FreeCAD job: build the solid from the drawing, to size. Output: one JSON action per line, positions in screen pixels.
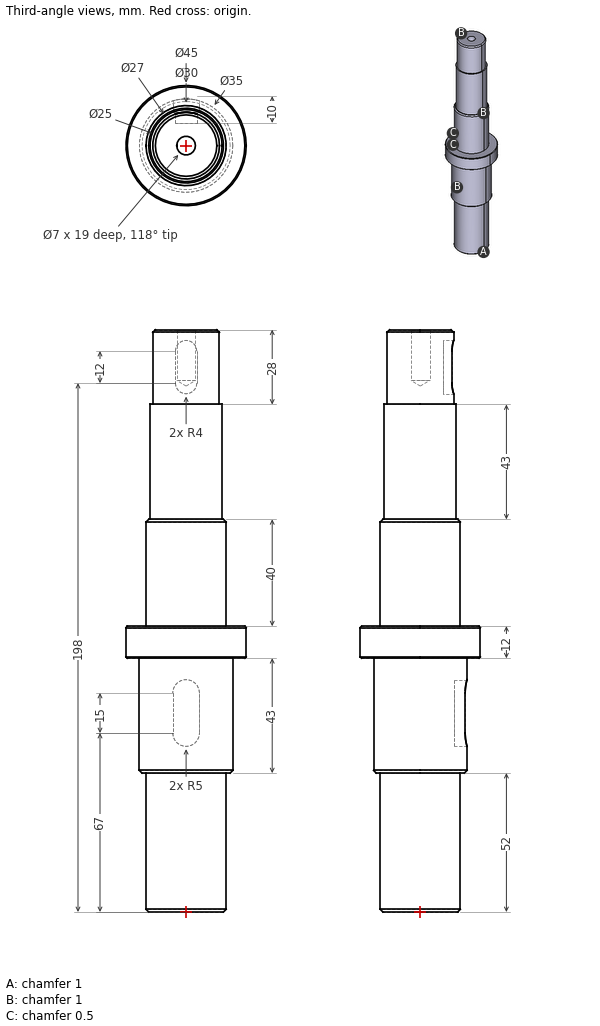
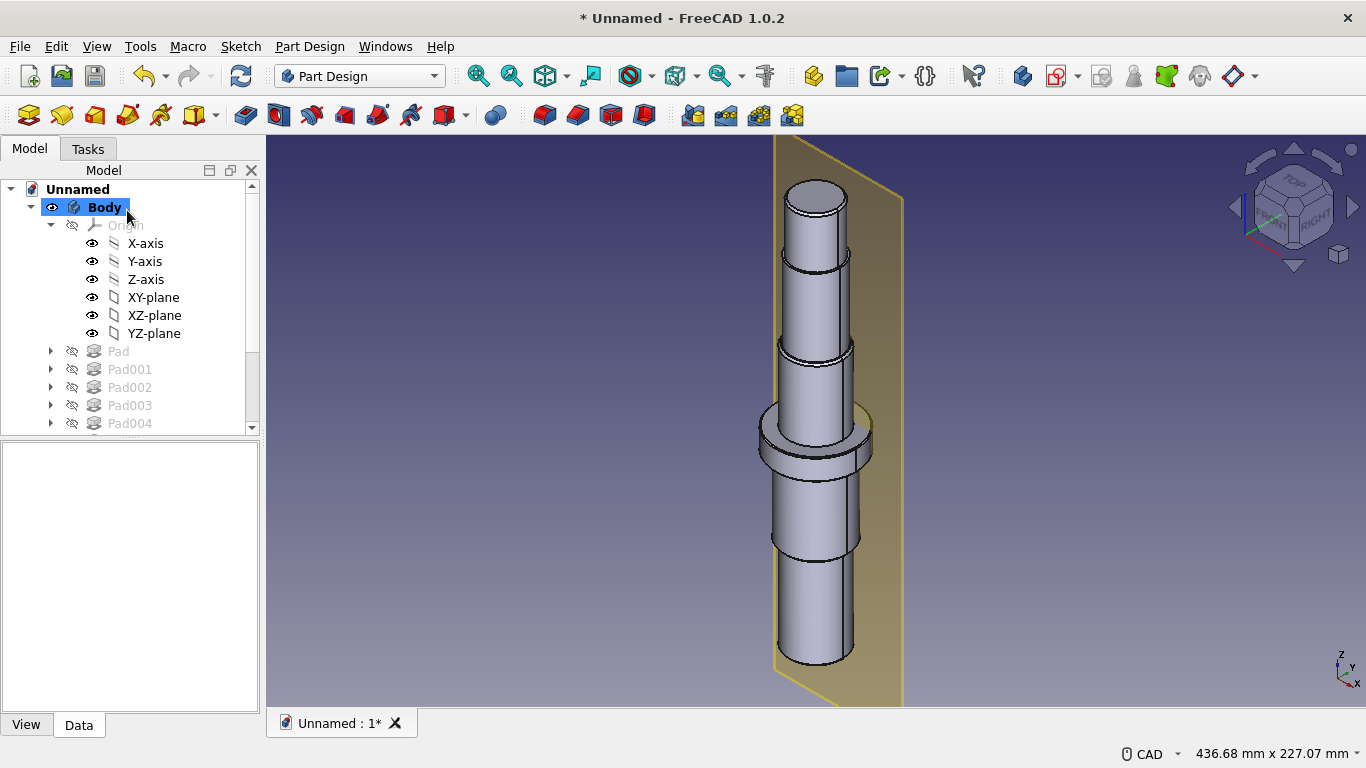
{"action": "scroll", "coordinate": [101, 311], "scroll_direction": "down", "scroll_amount": 3}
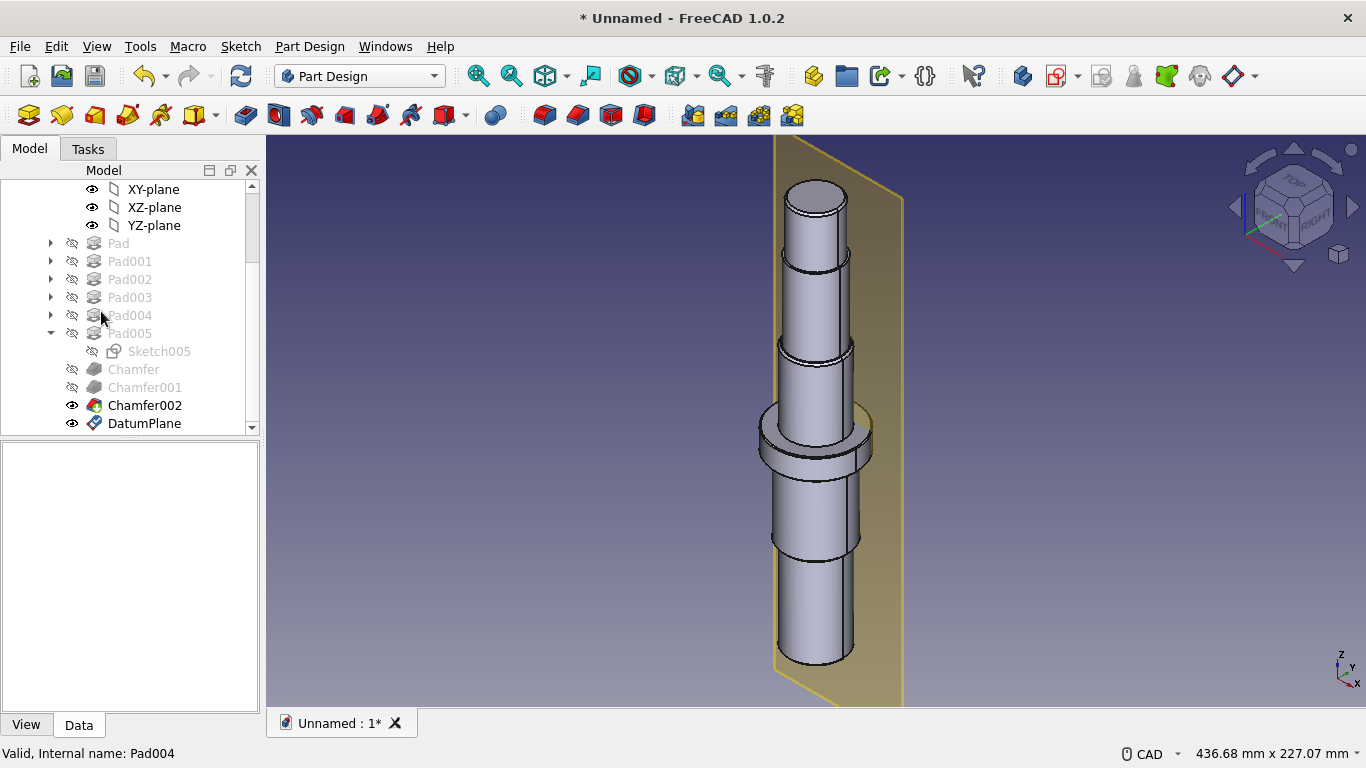
{"action": "left_click", "coordinate": [117, 423]}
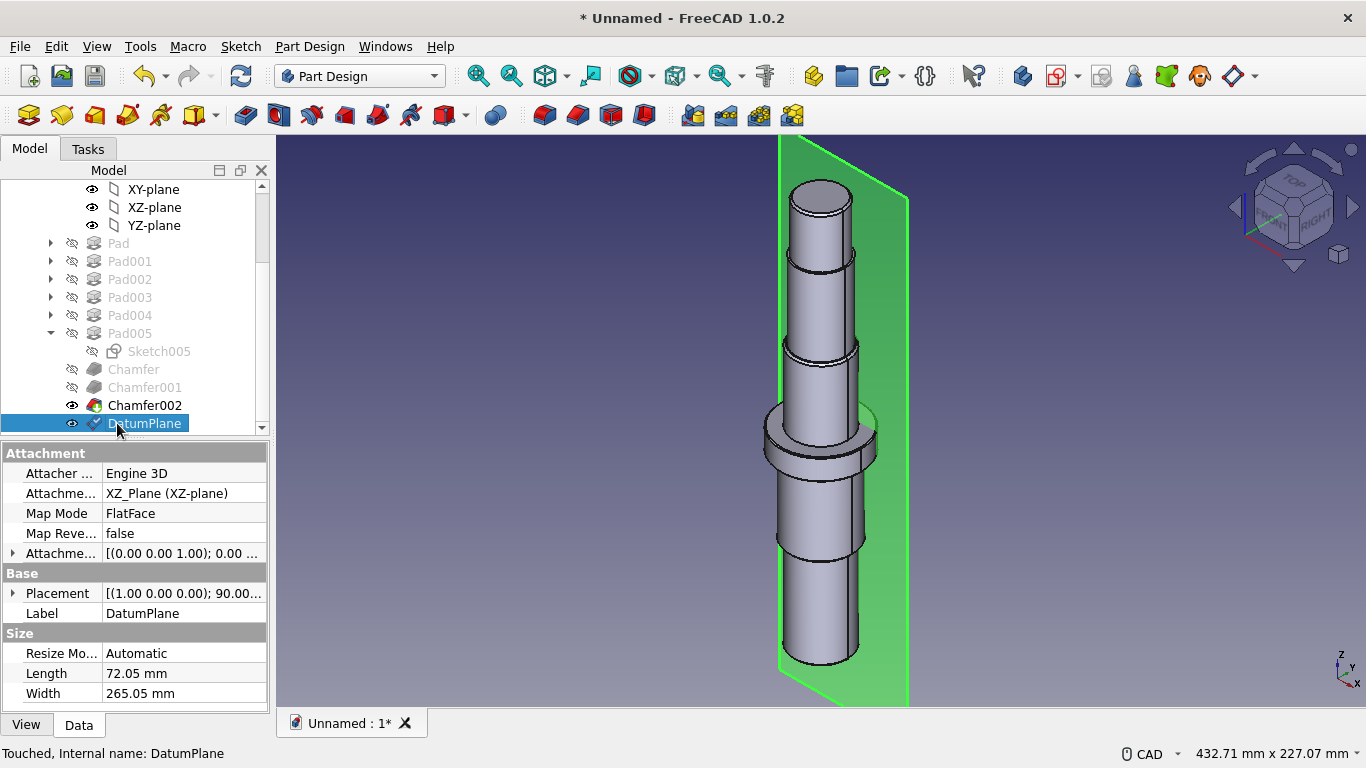
{"action": "left_click", "coordinate": [1056, 76]}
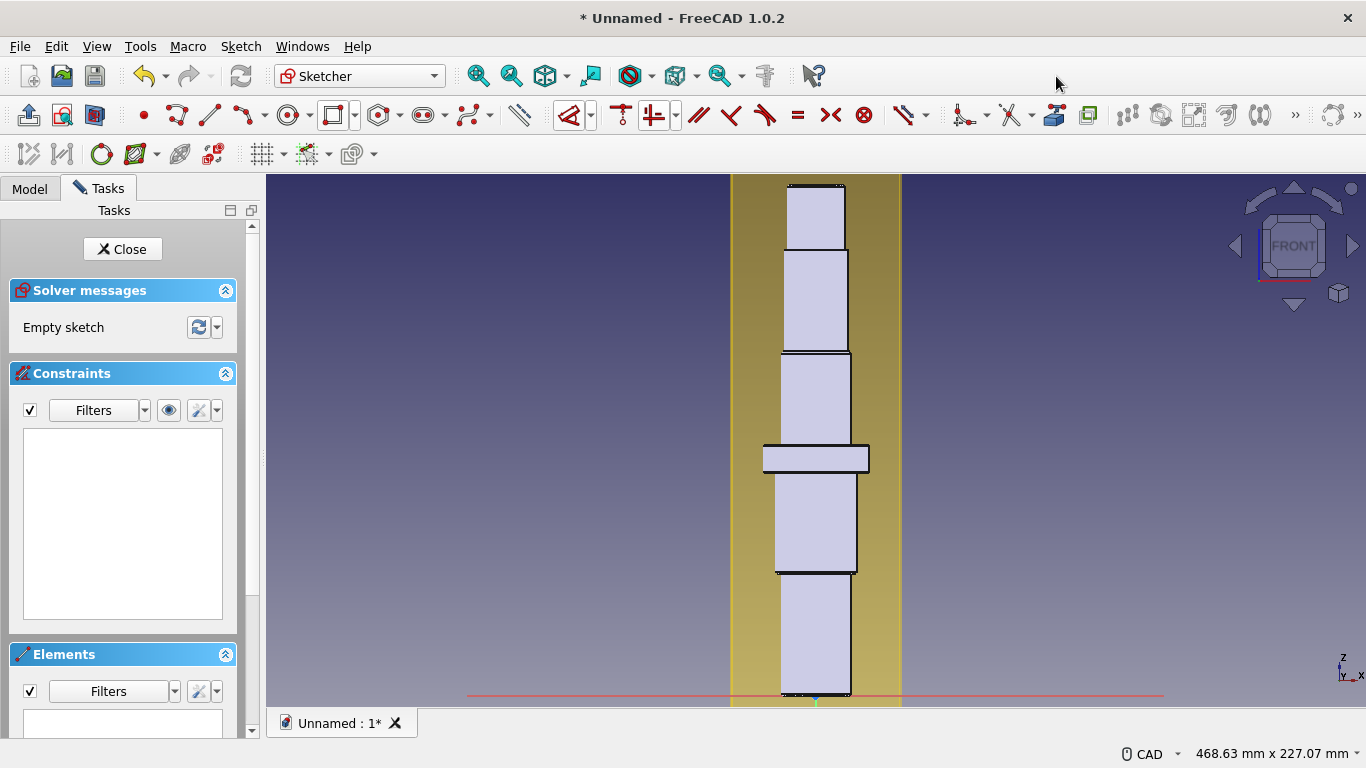
{"action": "left_click", "coordinate": [95, 116]}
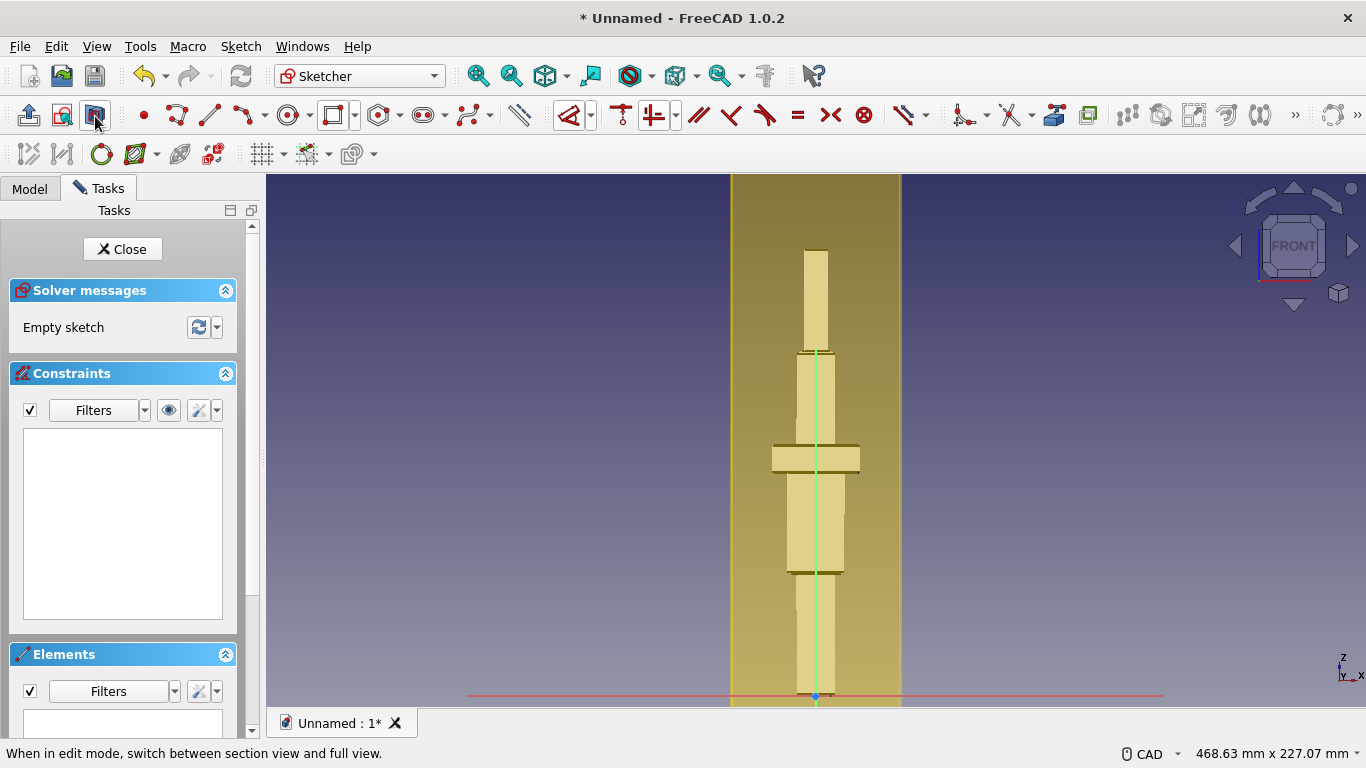
{"action": "scroll", "coordinate": [829, 538], "scroll_direction": "up", "scroll_amount": 9}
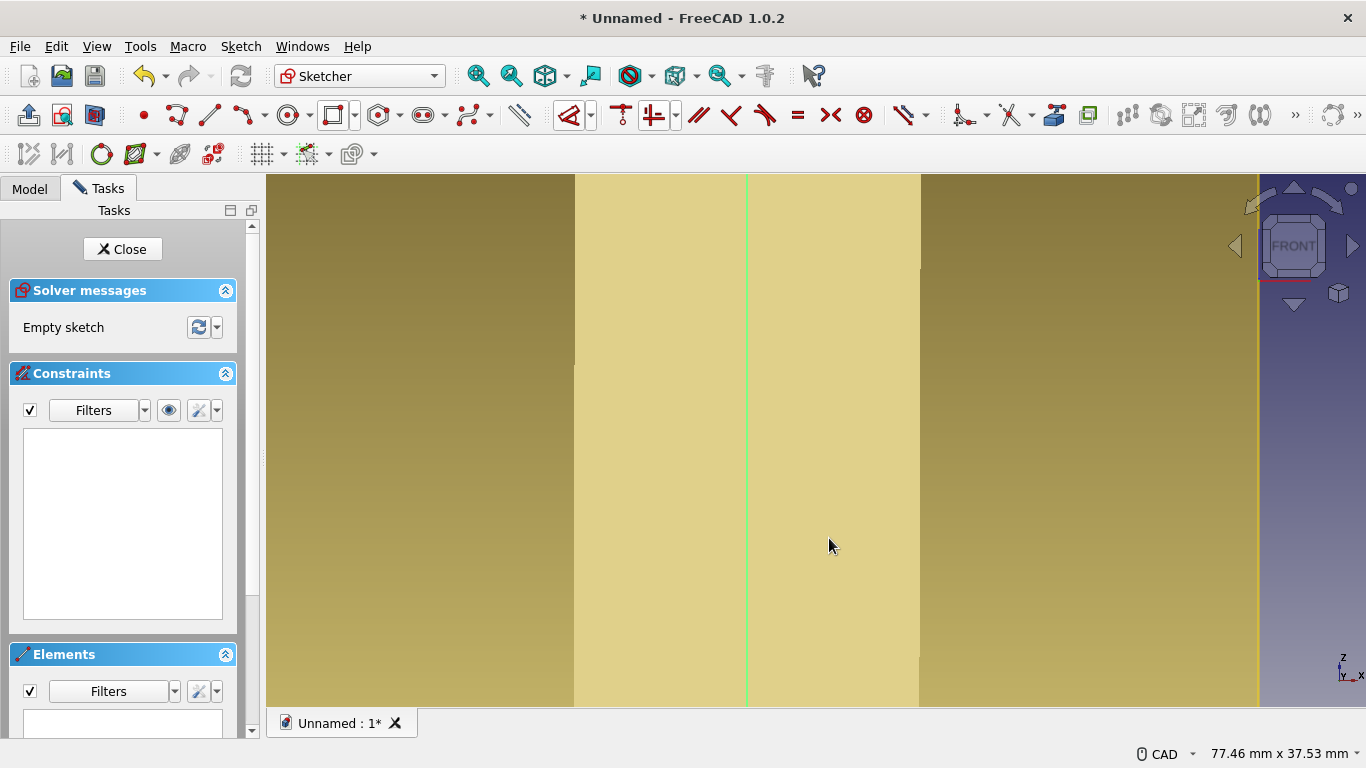
{"action": "left_click", "coordinate": [422, 116]}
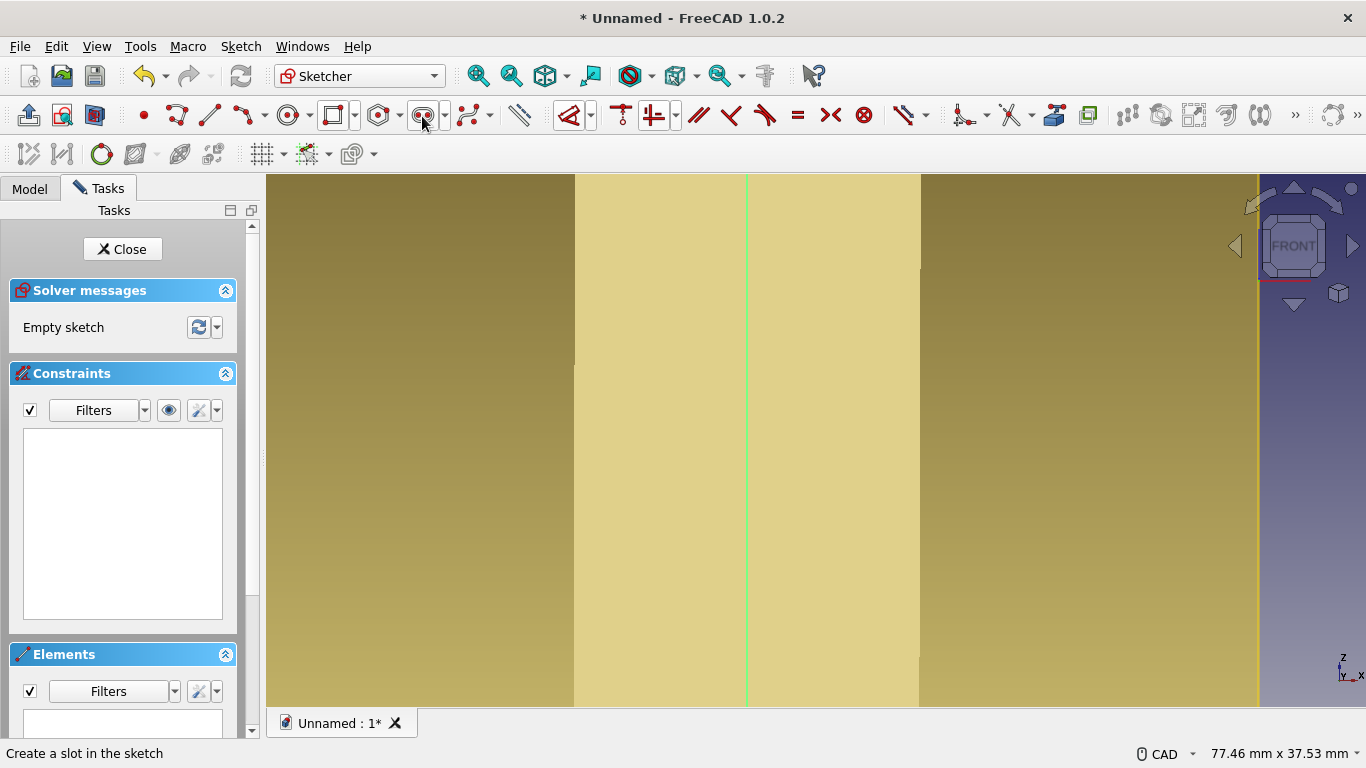
{"action": "left_click", "coordinate": [747, 541]}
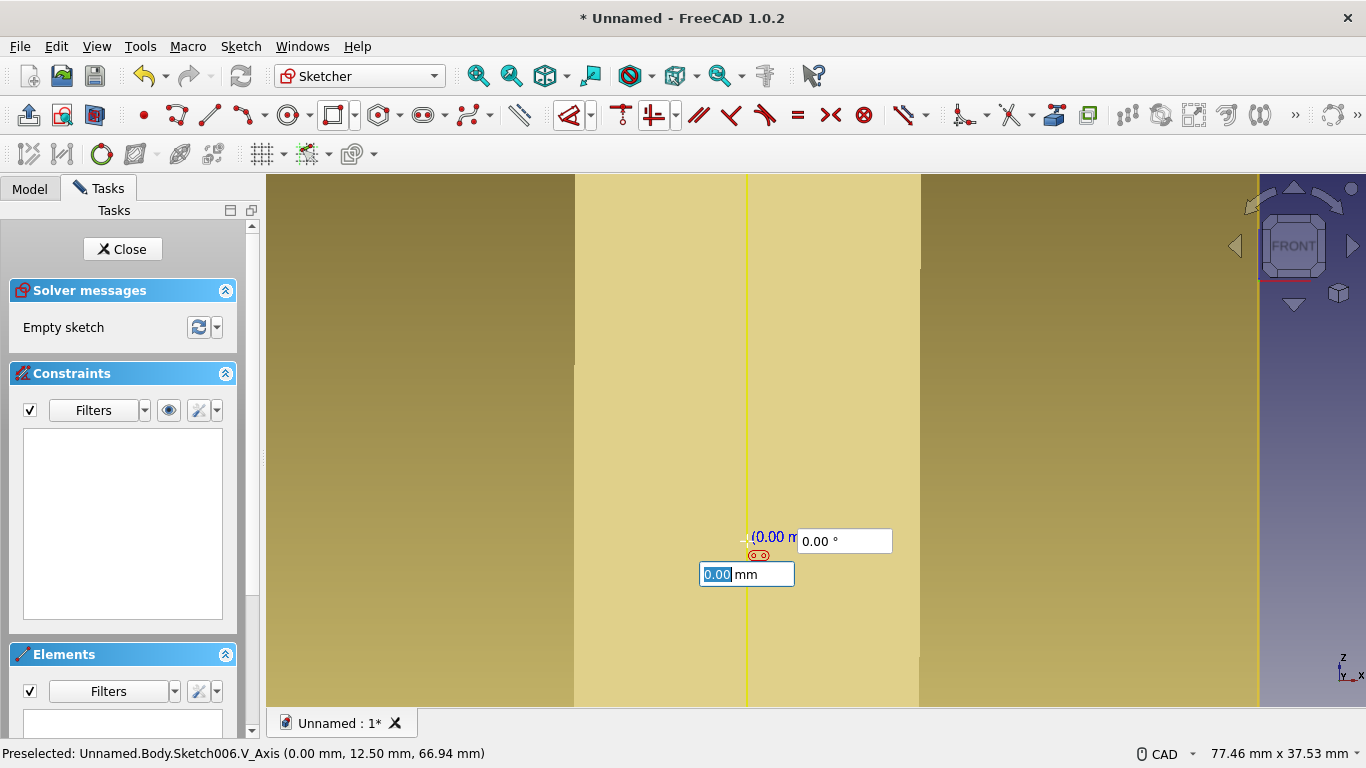
{"action": "left_click", "coordinate": [756, 328]}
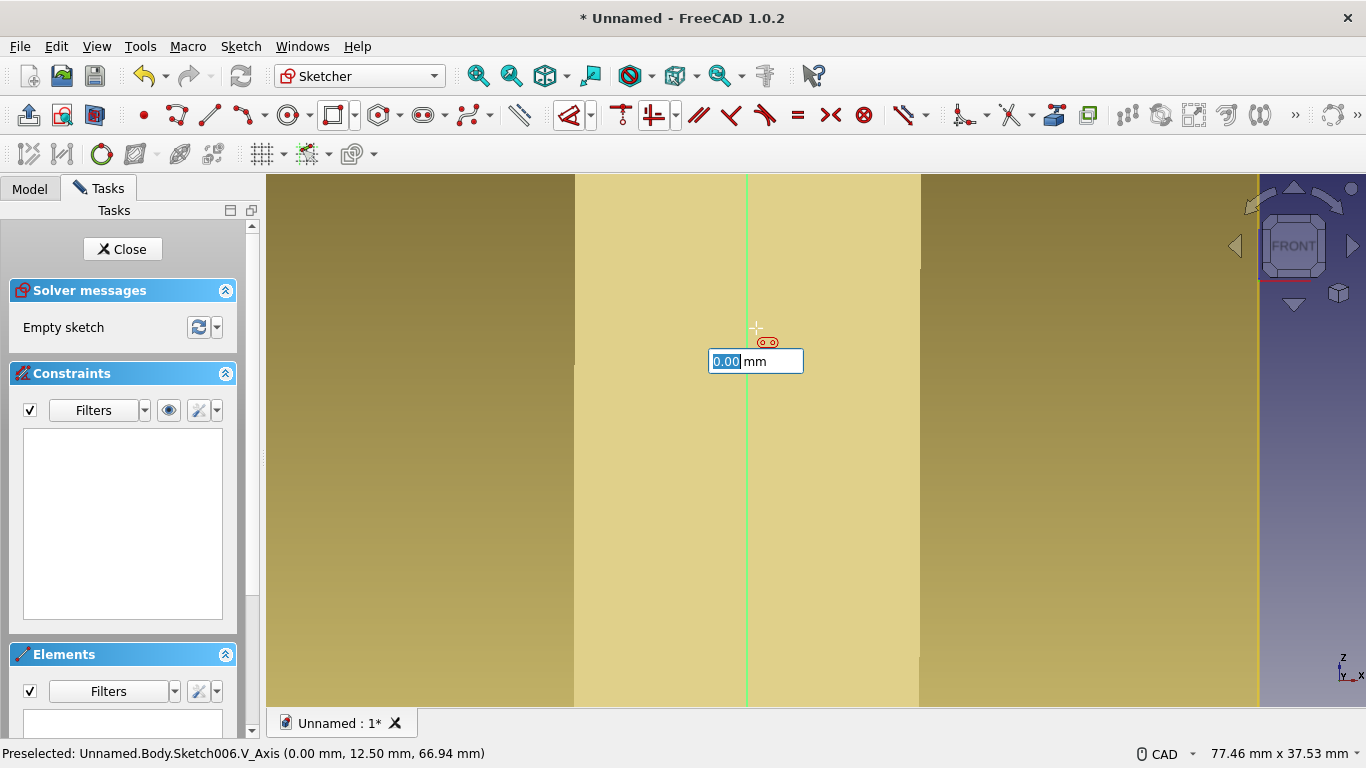
{"action": "left_click", "coordinate": [818, 435]}
{"action": "key", "text": "Escape"}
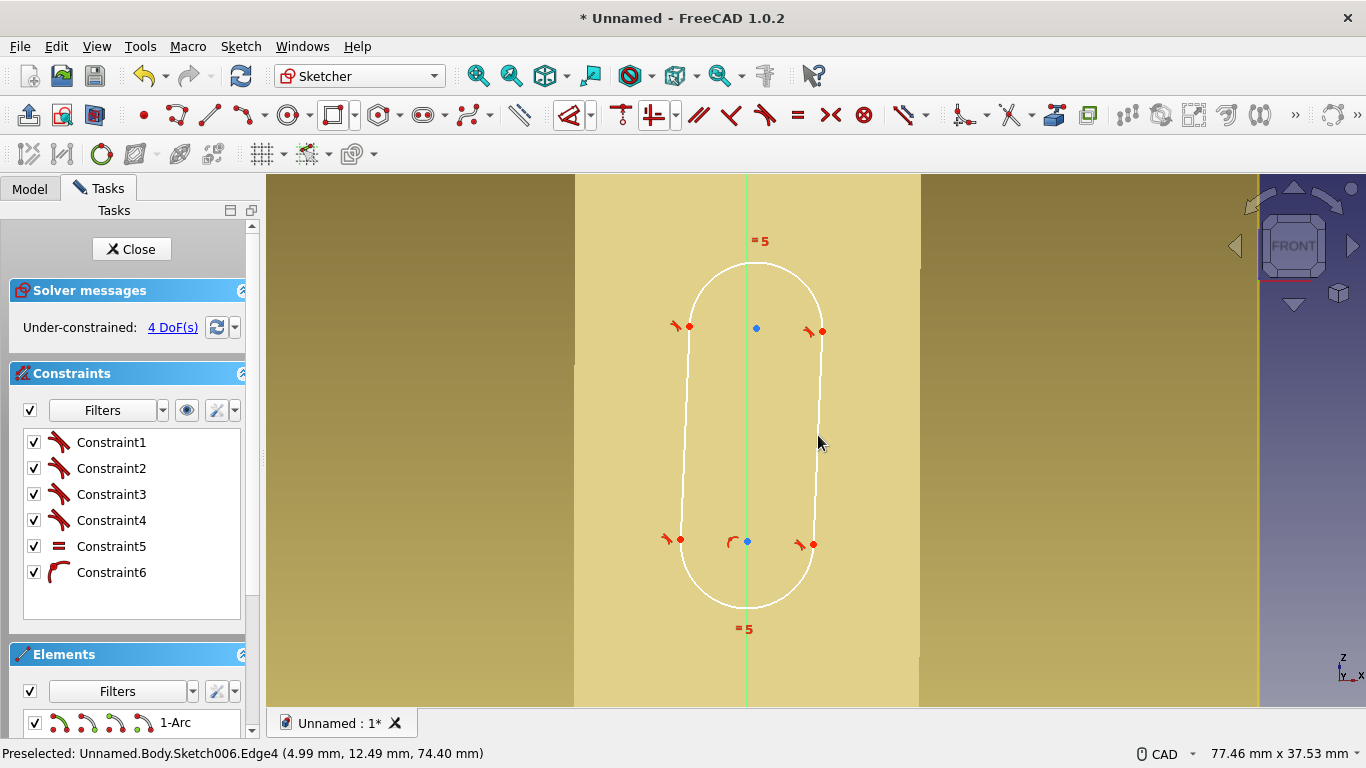
{"action": "left_click", "coordinate": [683, 475]}